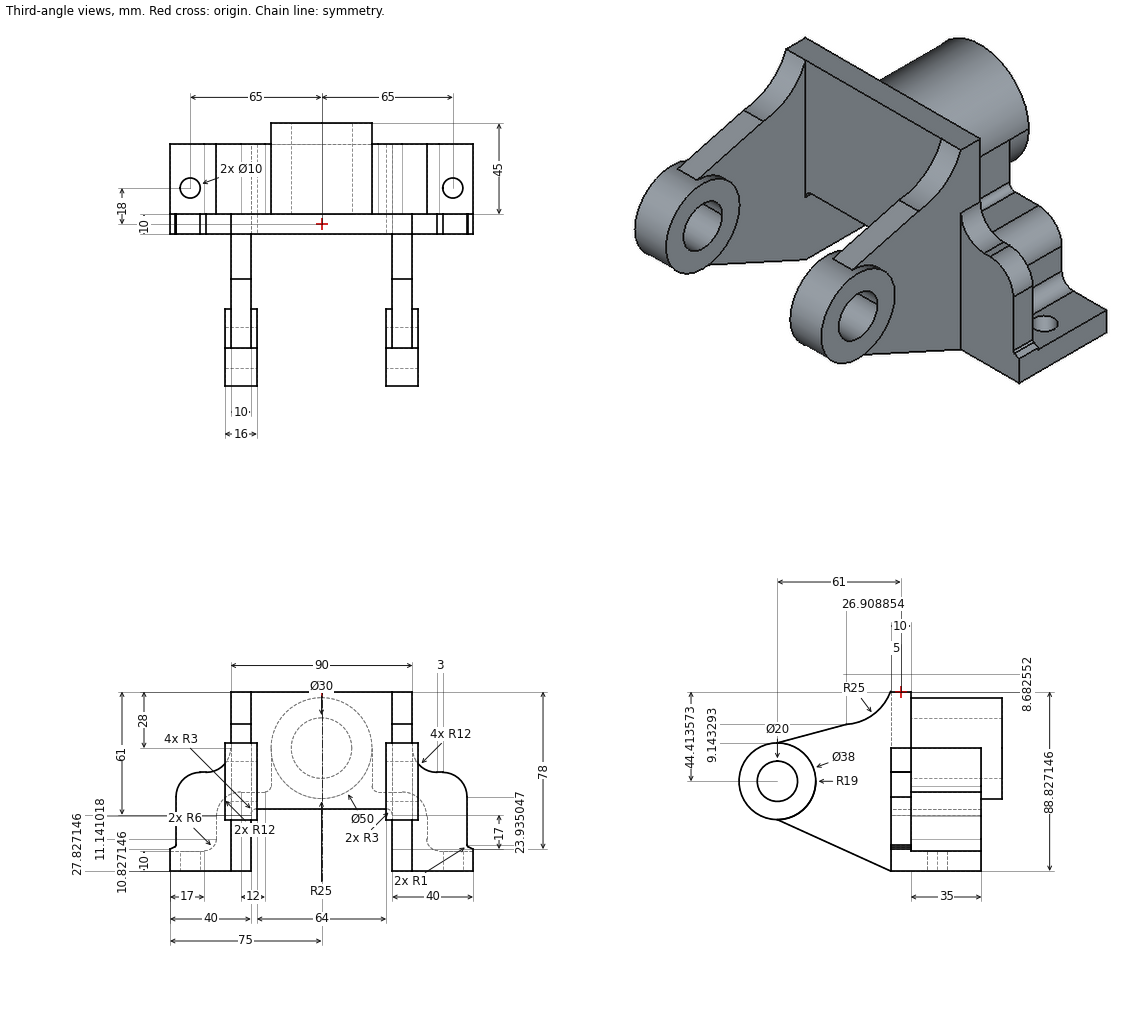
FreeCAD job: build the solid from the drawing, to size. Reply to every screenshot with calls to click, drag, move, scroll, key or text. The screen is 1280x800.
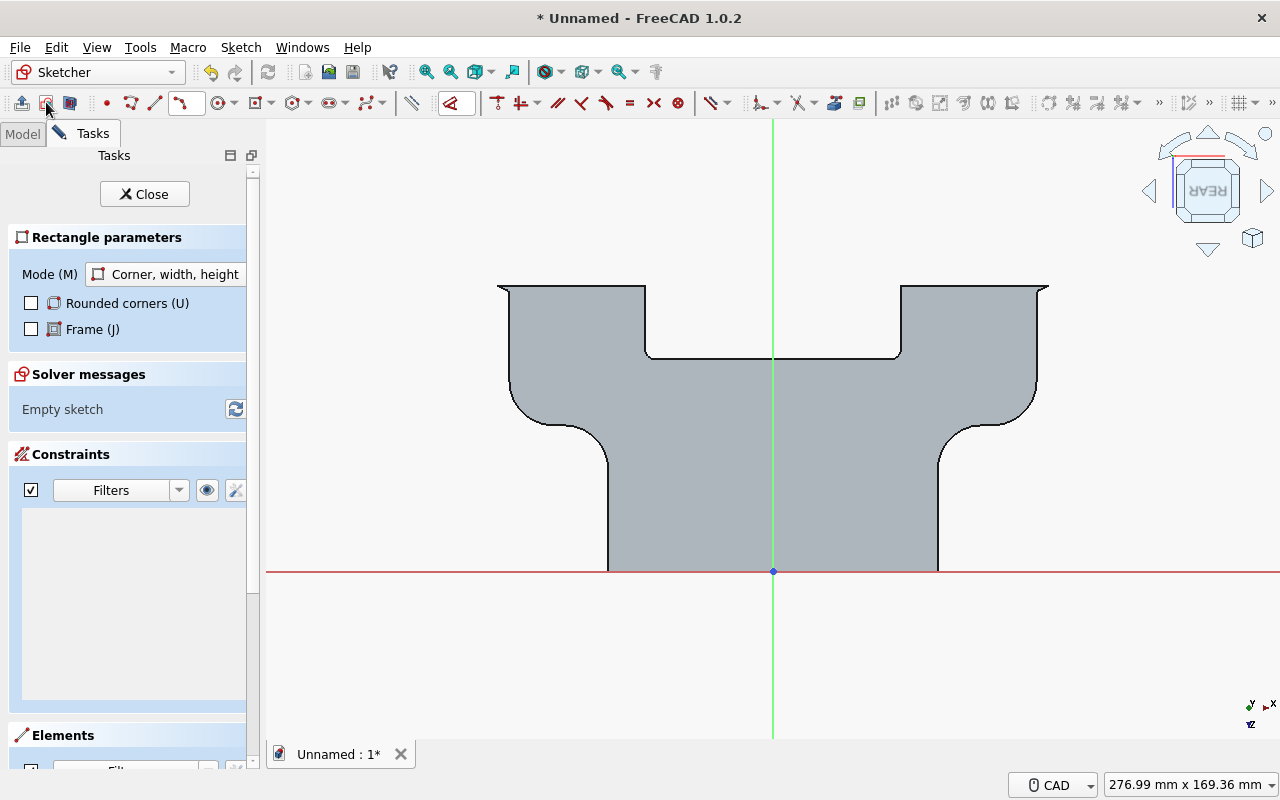
click(498, 247)
click(645, 286)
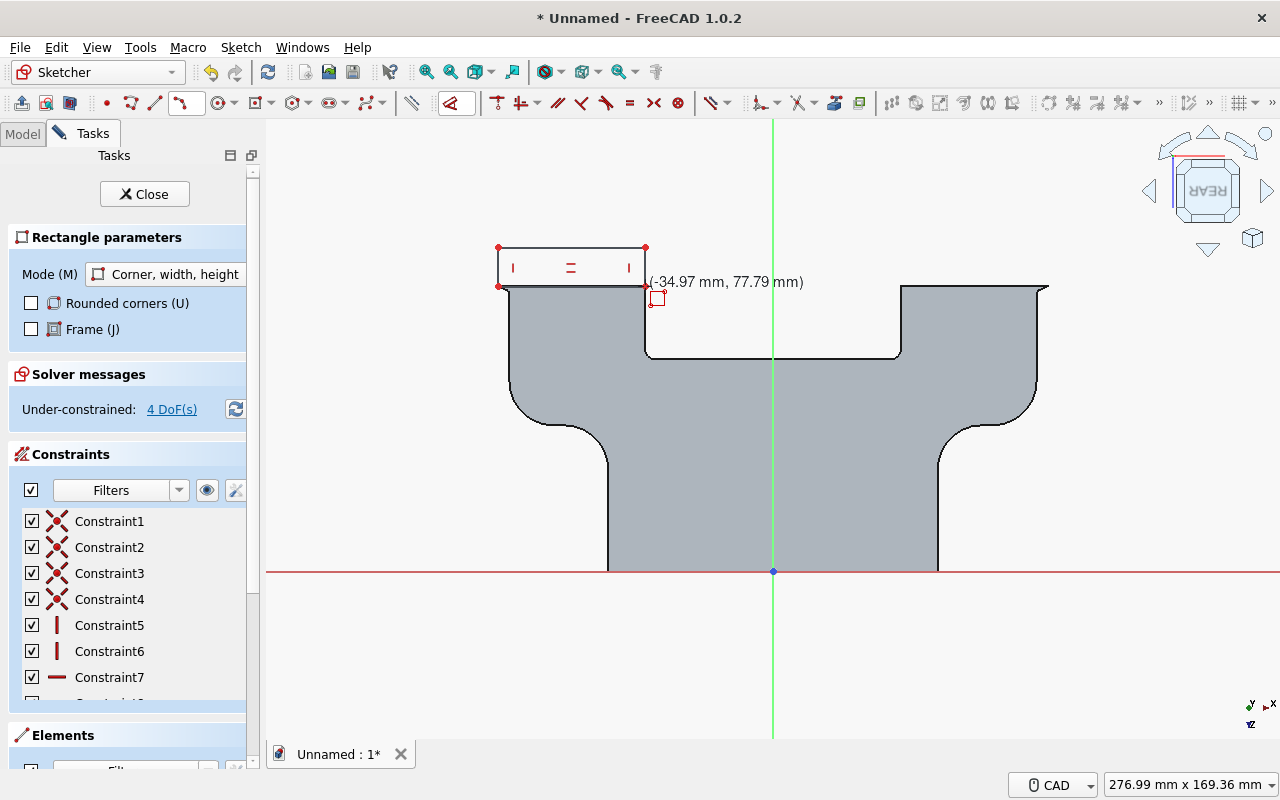
click(901, 247)
click(1048, 286)
key(Escape)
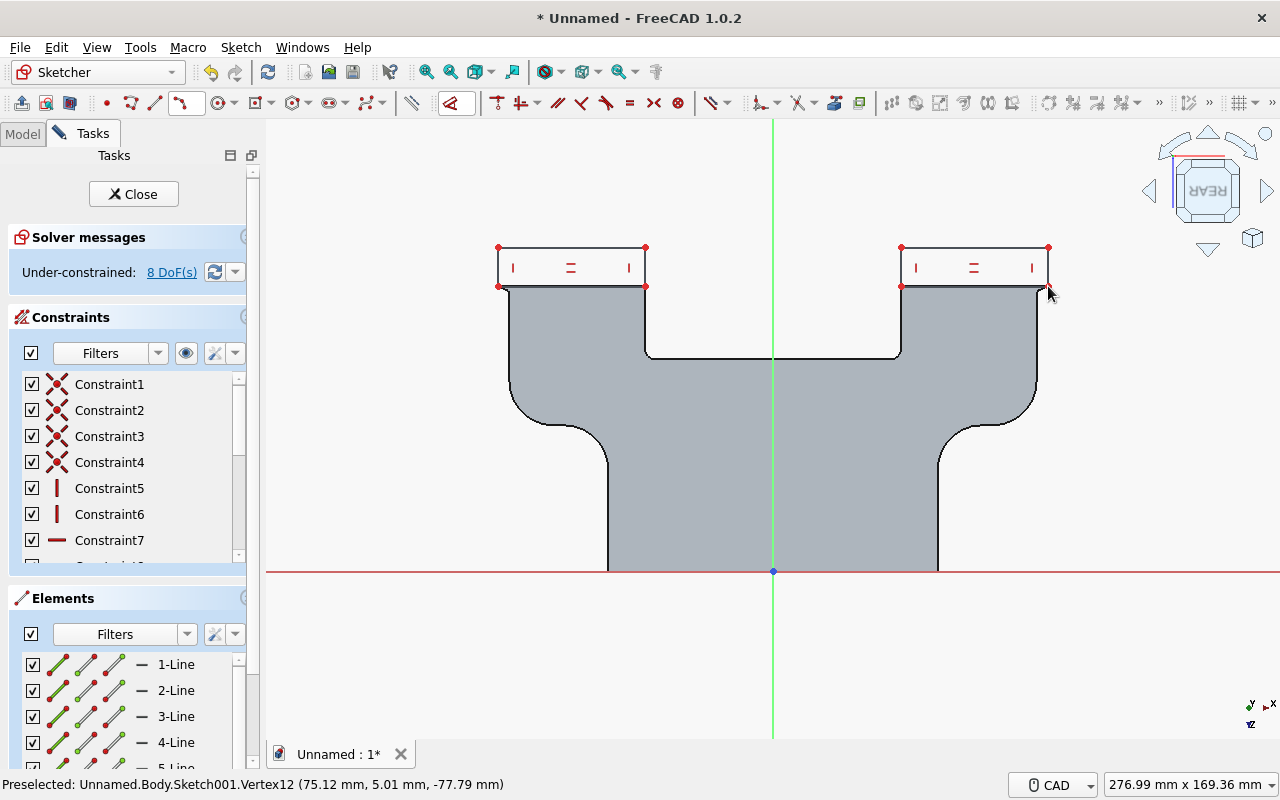
click(645, 248)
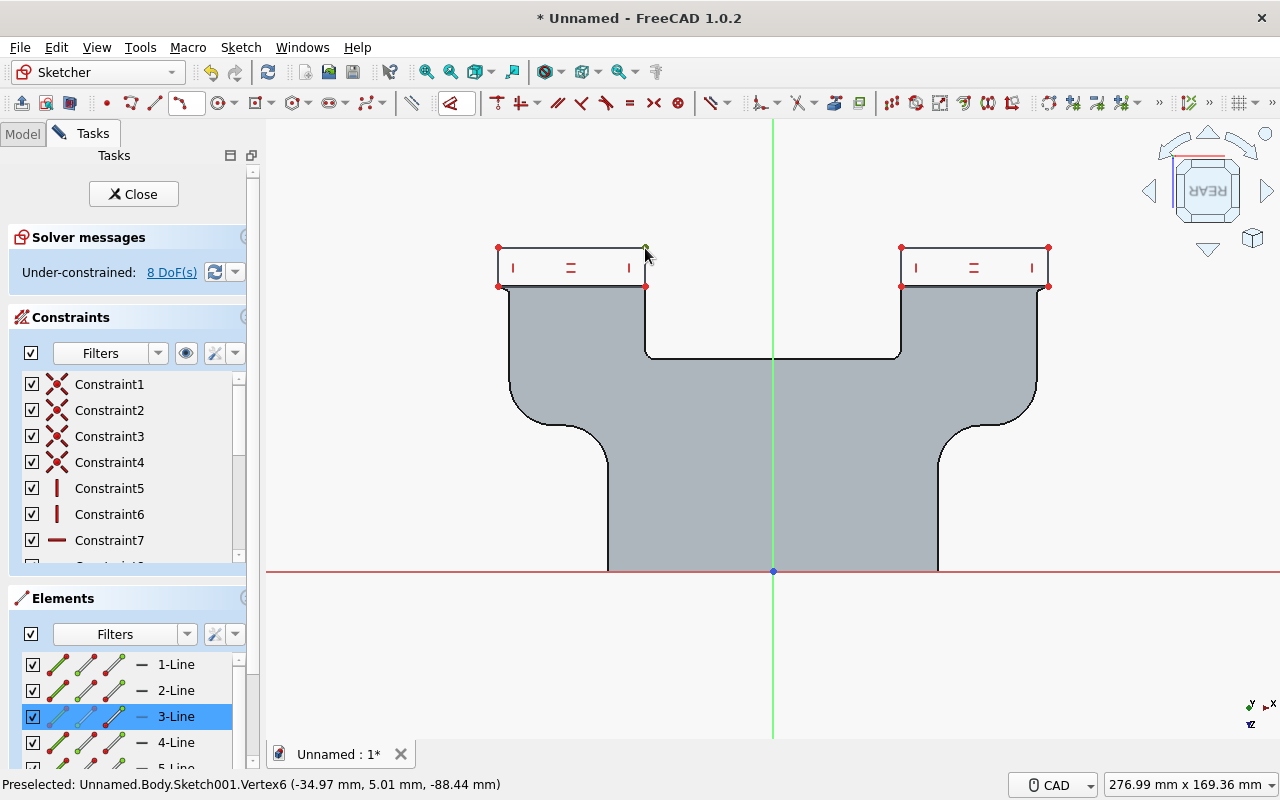
click(901, 248)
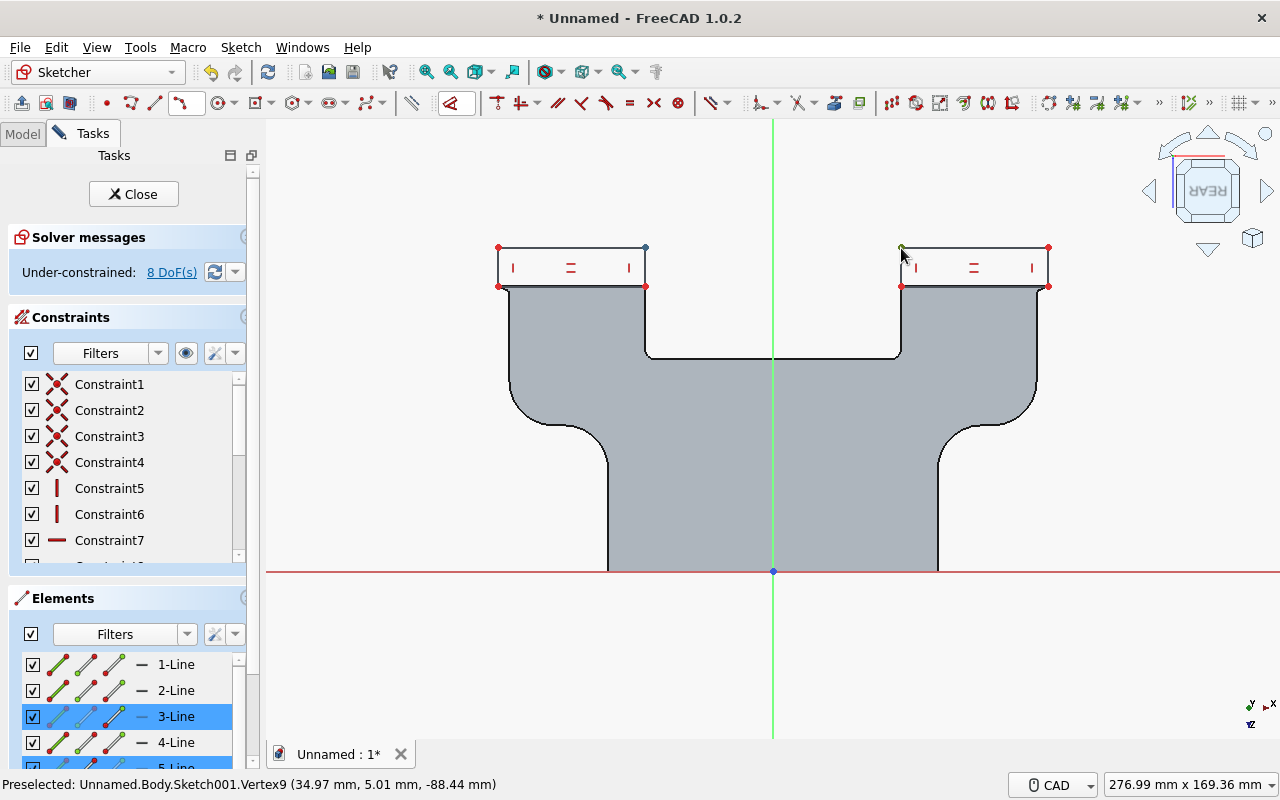
click(773, 671)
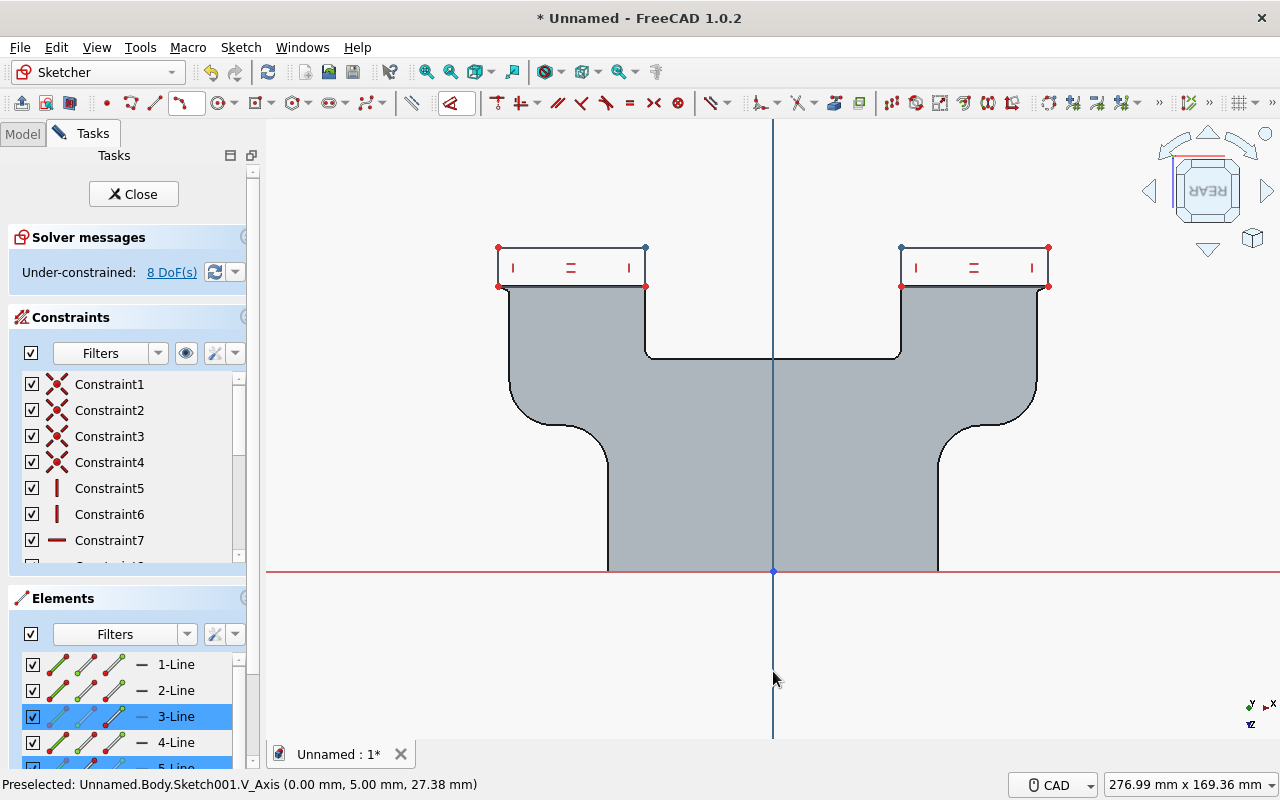
click(654, 104)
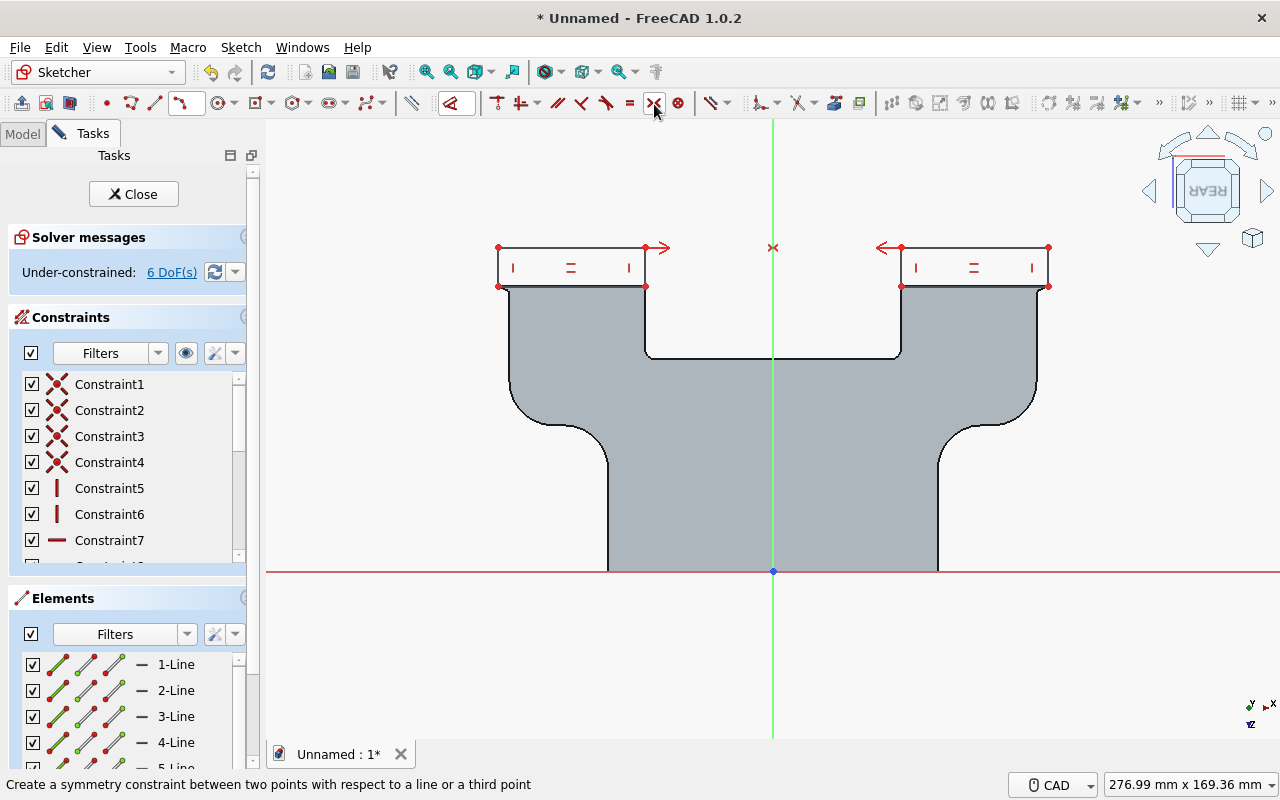
click(498, 287)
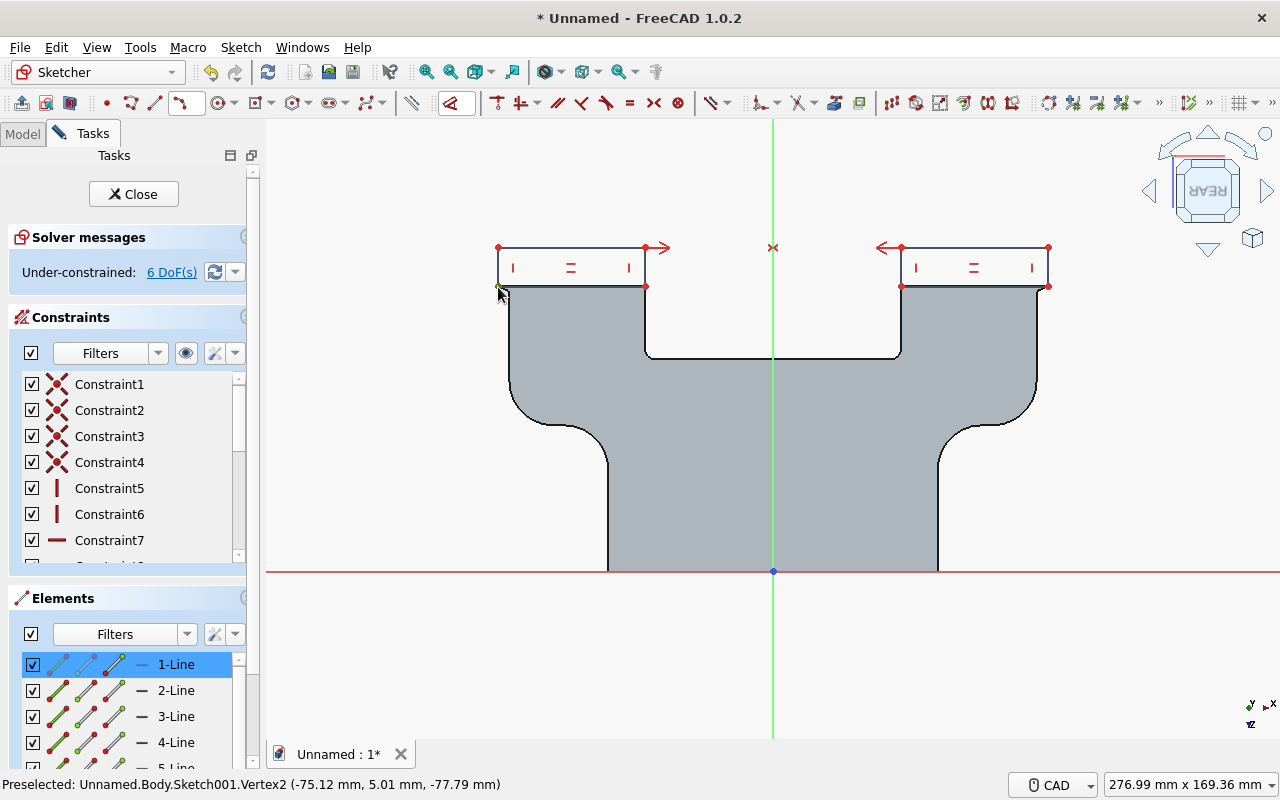
click(1048, 287)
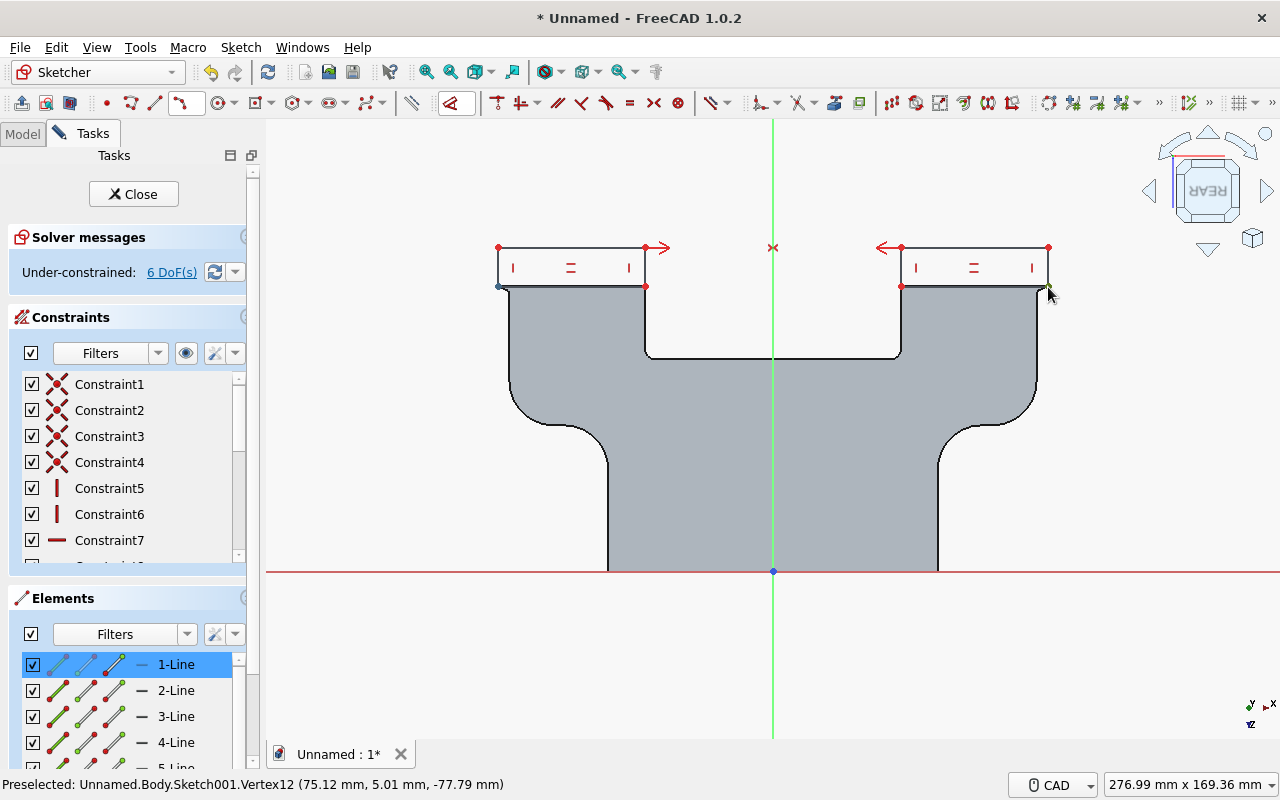
click(773, 671)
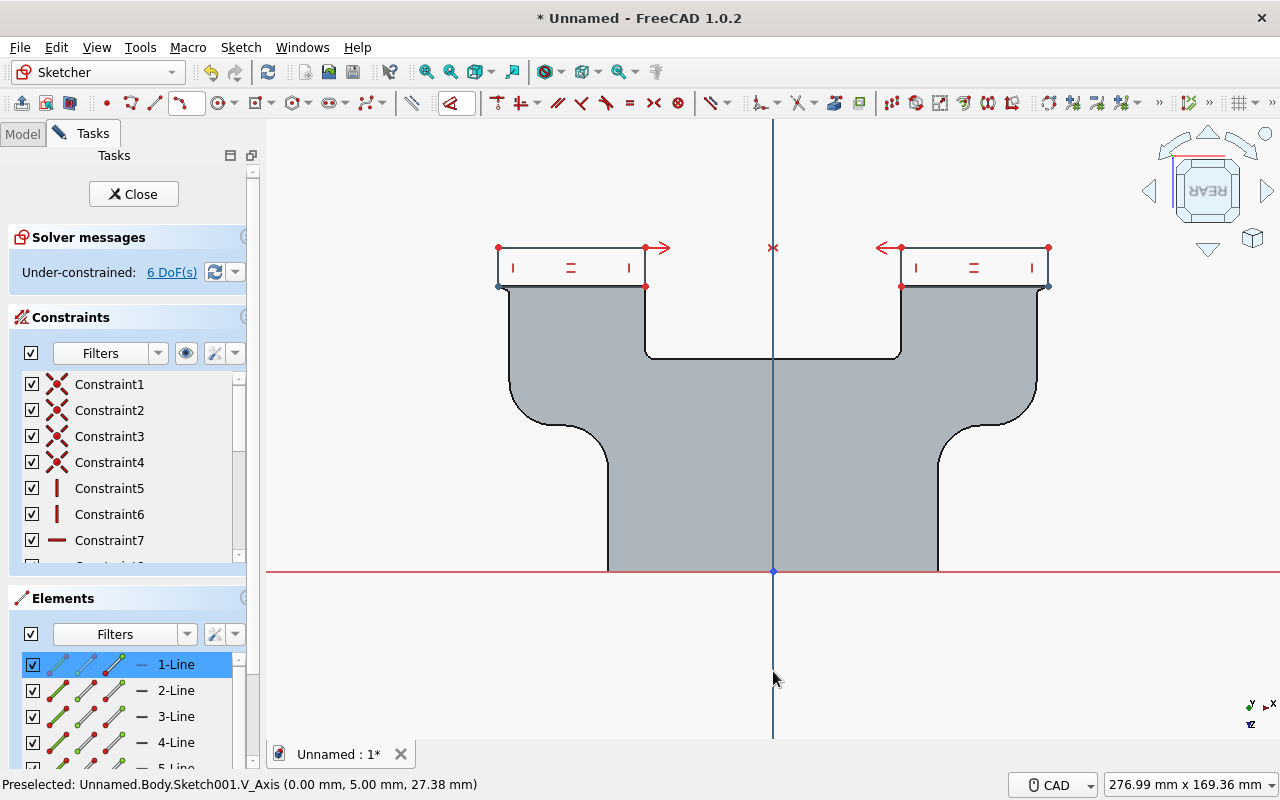
click(654, 104)